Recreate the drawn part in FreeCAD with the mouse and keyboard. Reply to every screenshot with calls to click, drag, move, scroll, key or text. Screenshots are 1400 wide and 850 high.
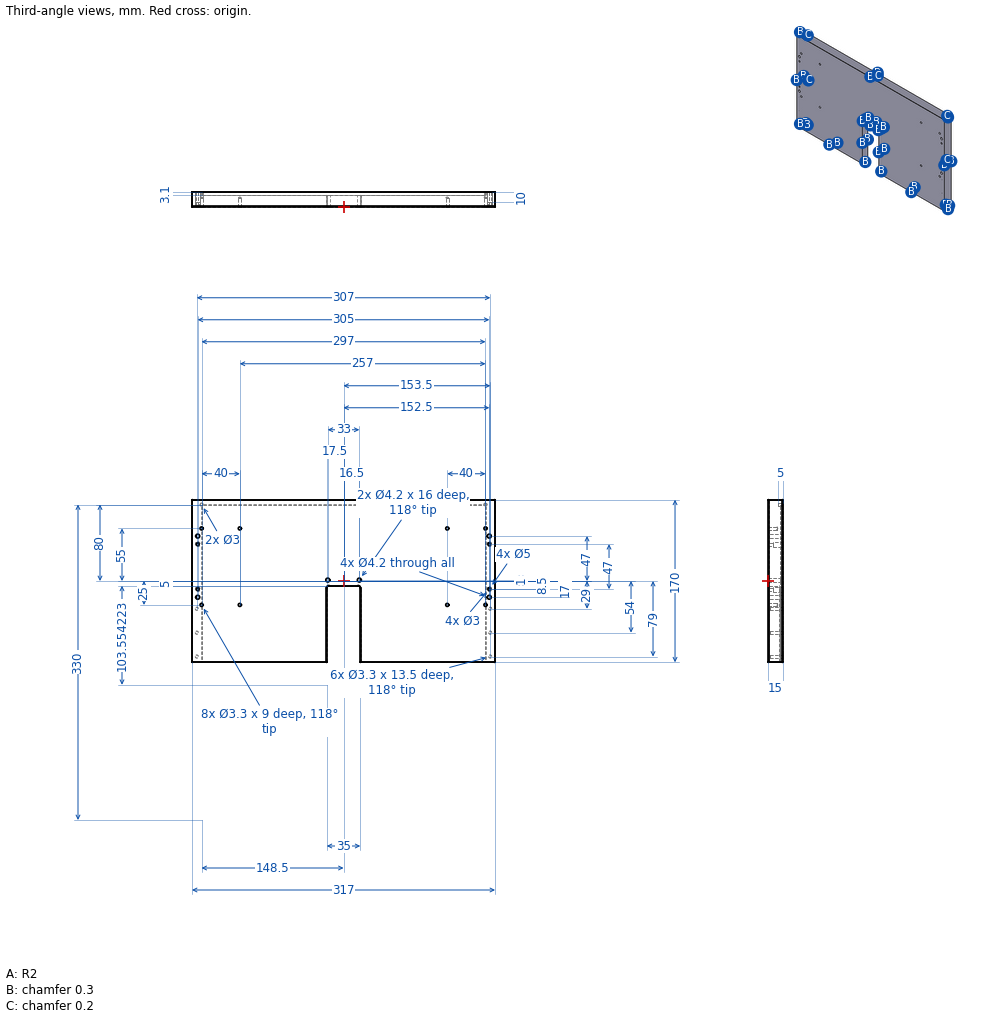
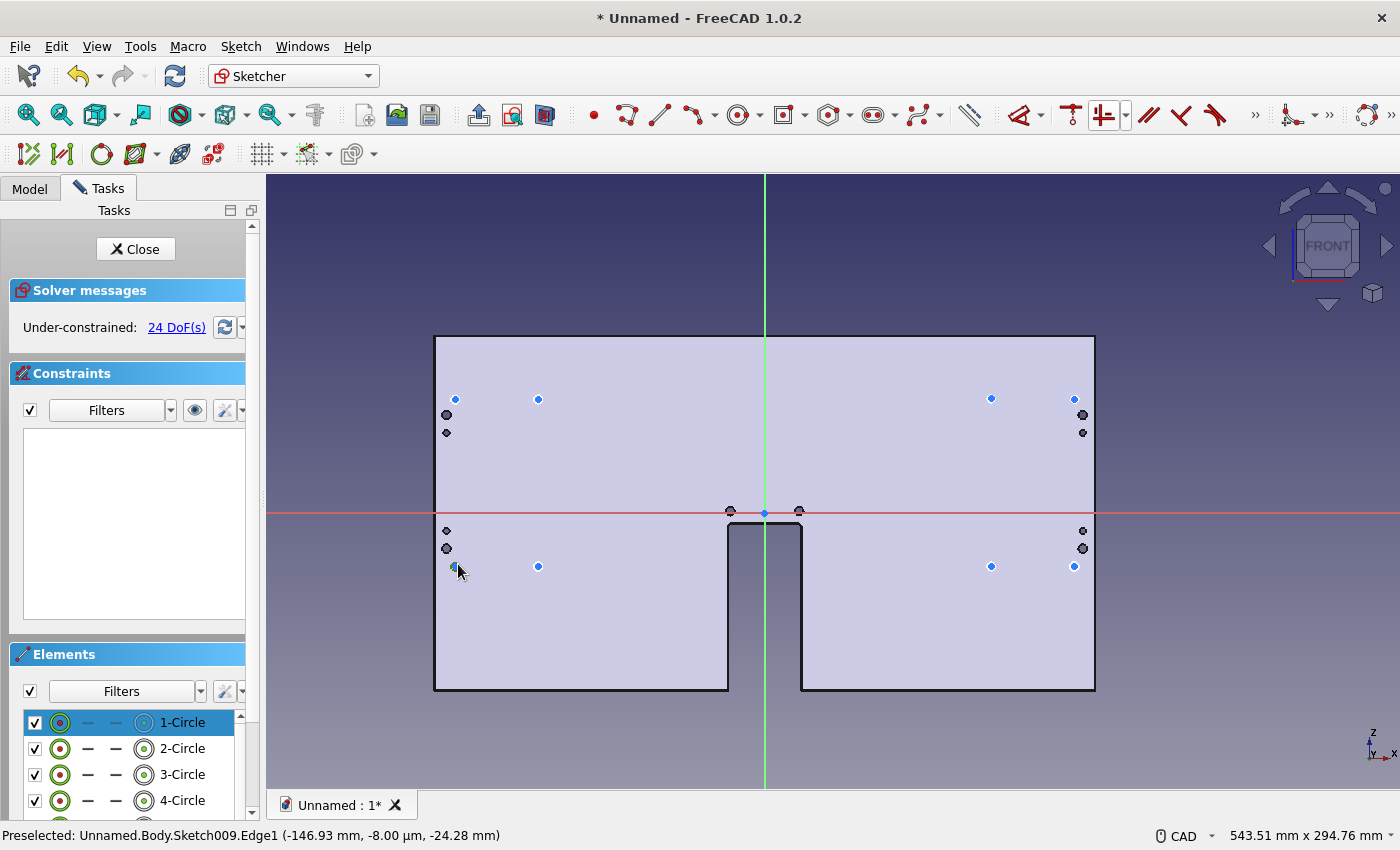
scroll(458, 397, up, 7)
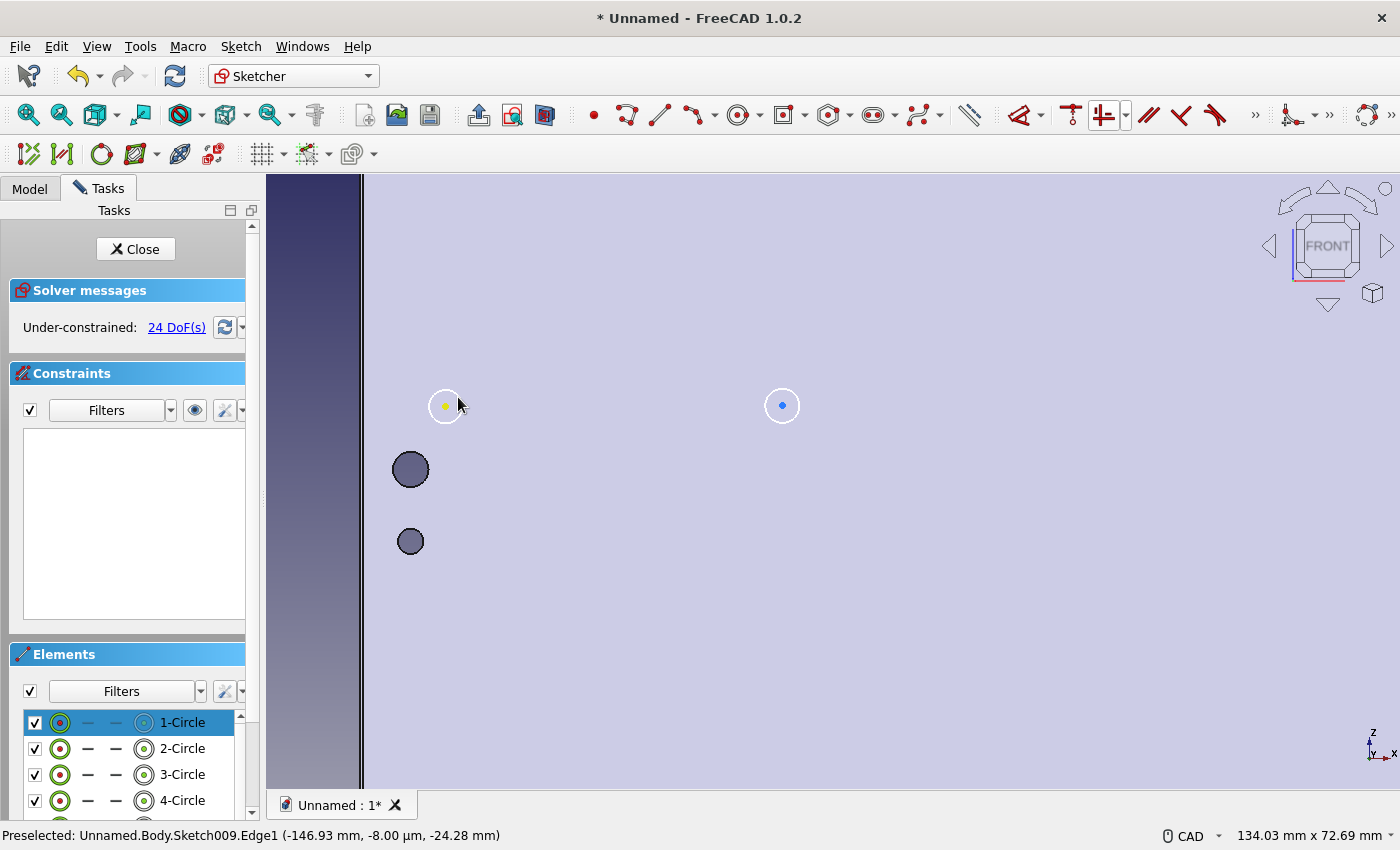
click(458, 395)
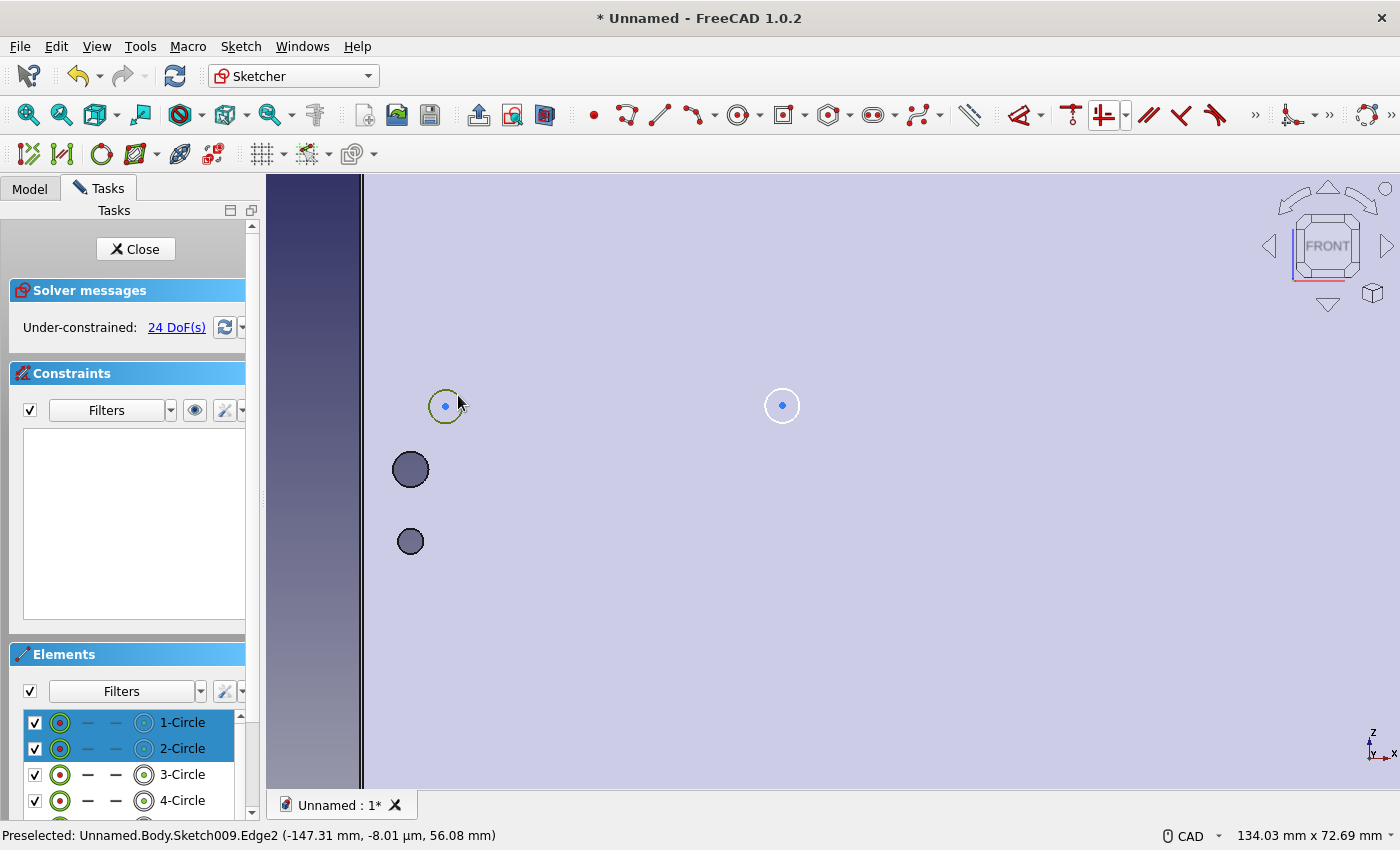
scroll(458, 397, down, 7)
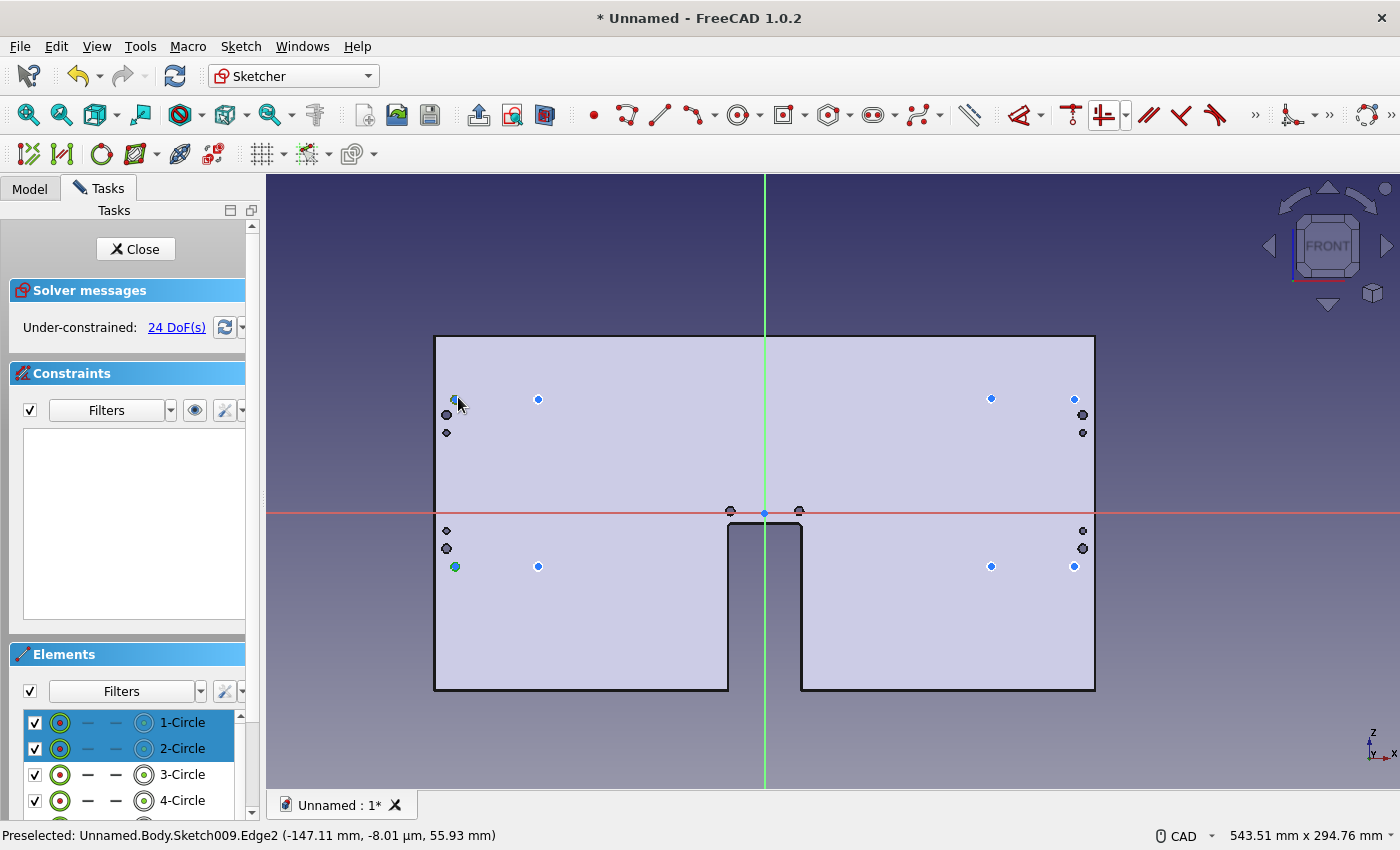
scroll(541, 564, up, 6)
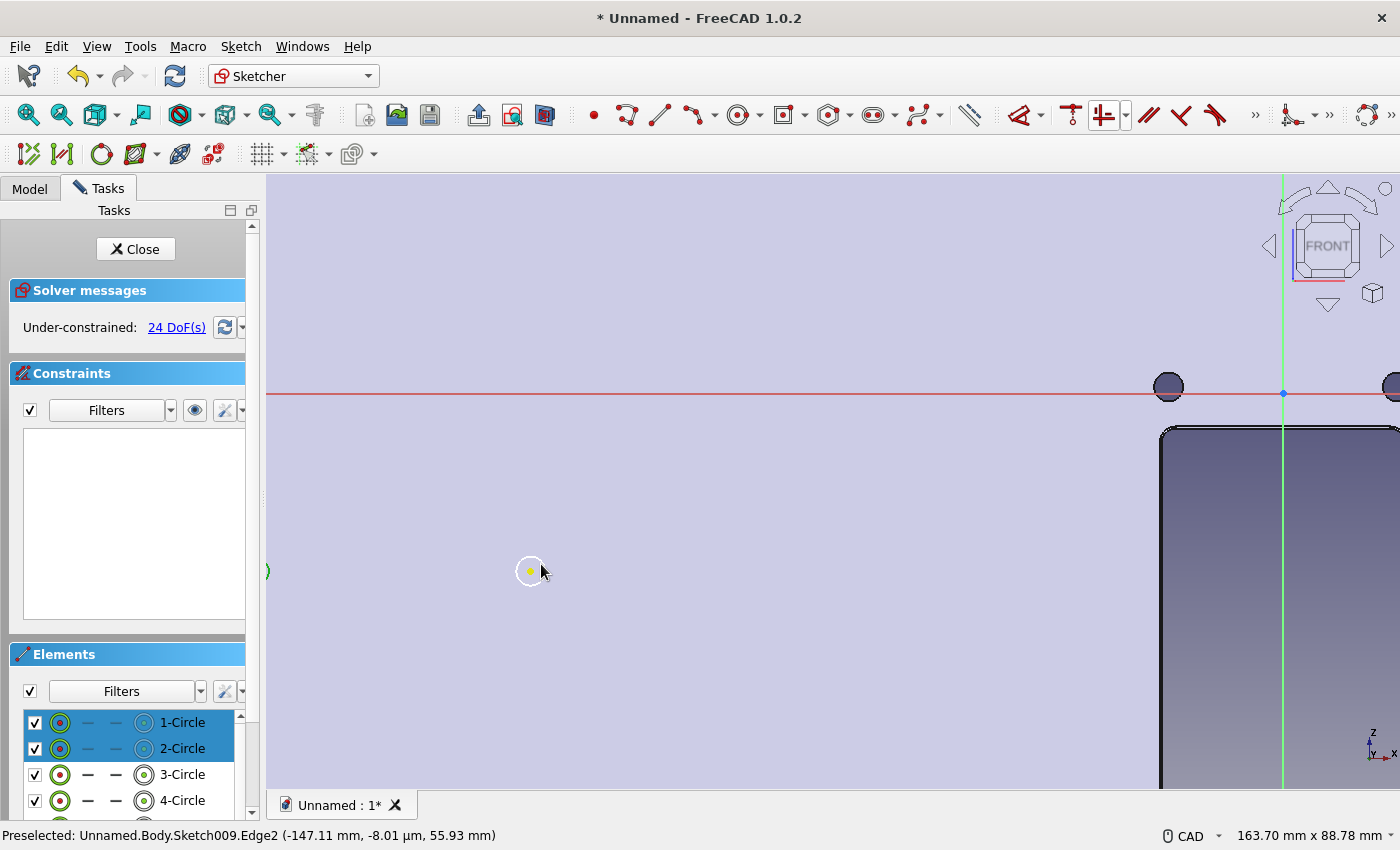
click(541, 561)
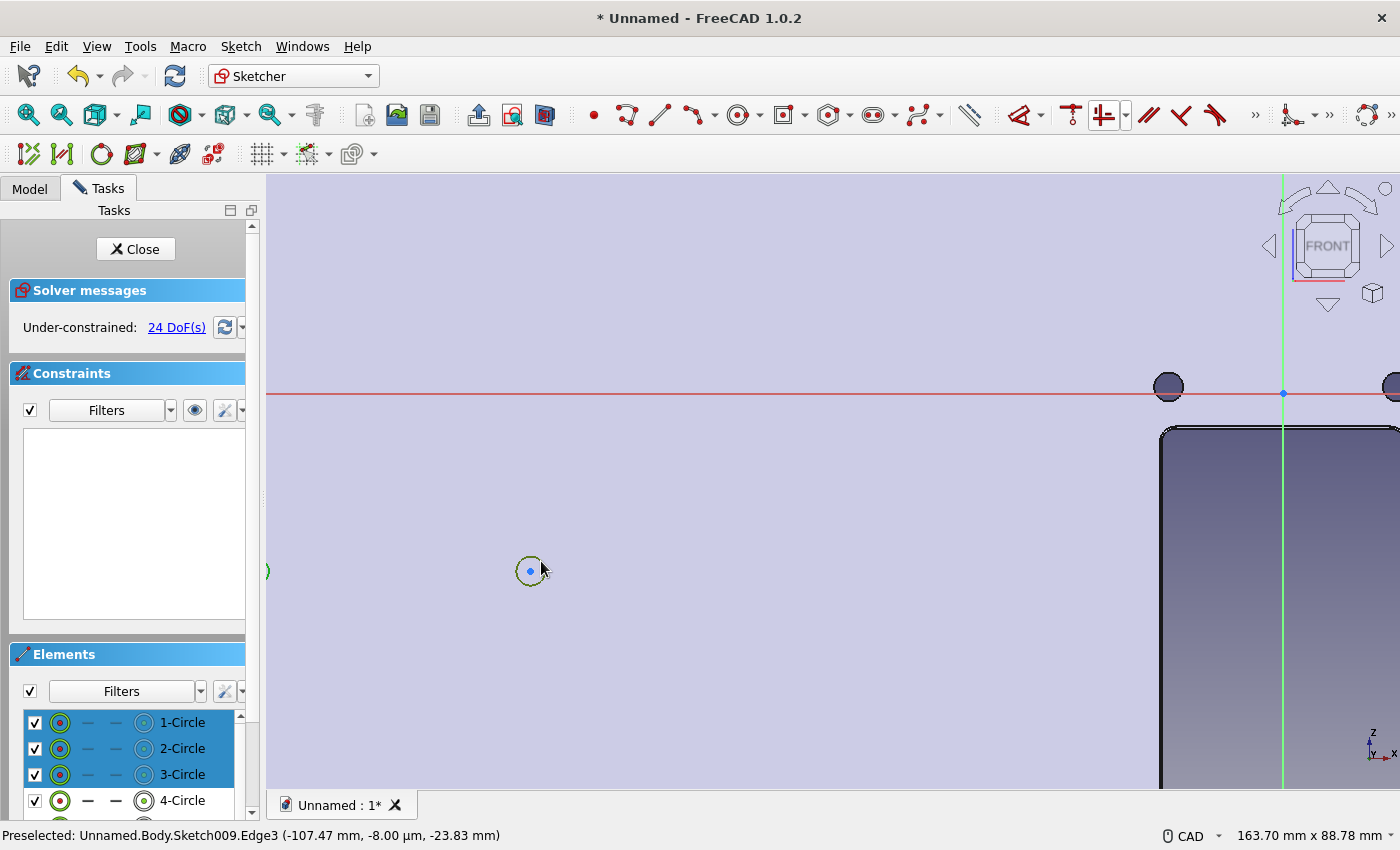
scroll(541, 564, down, 6)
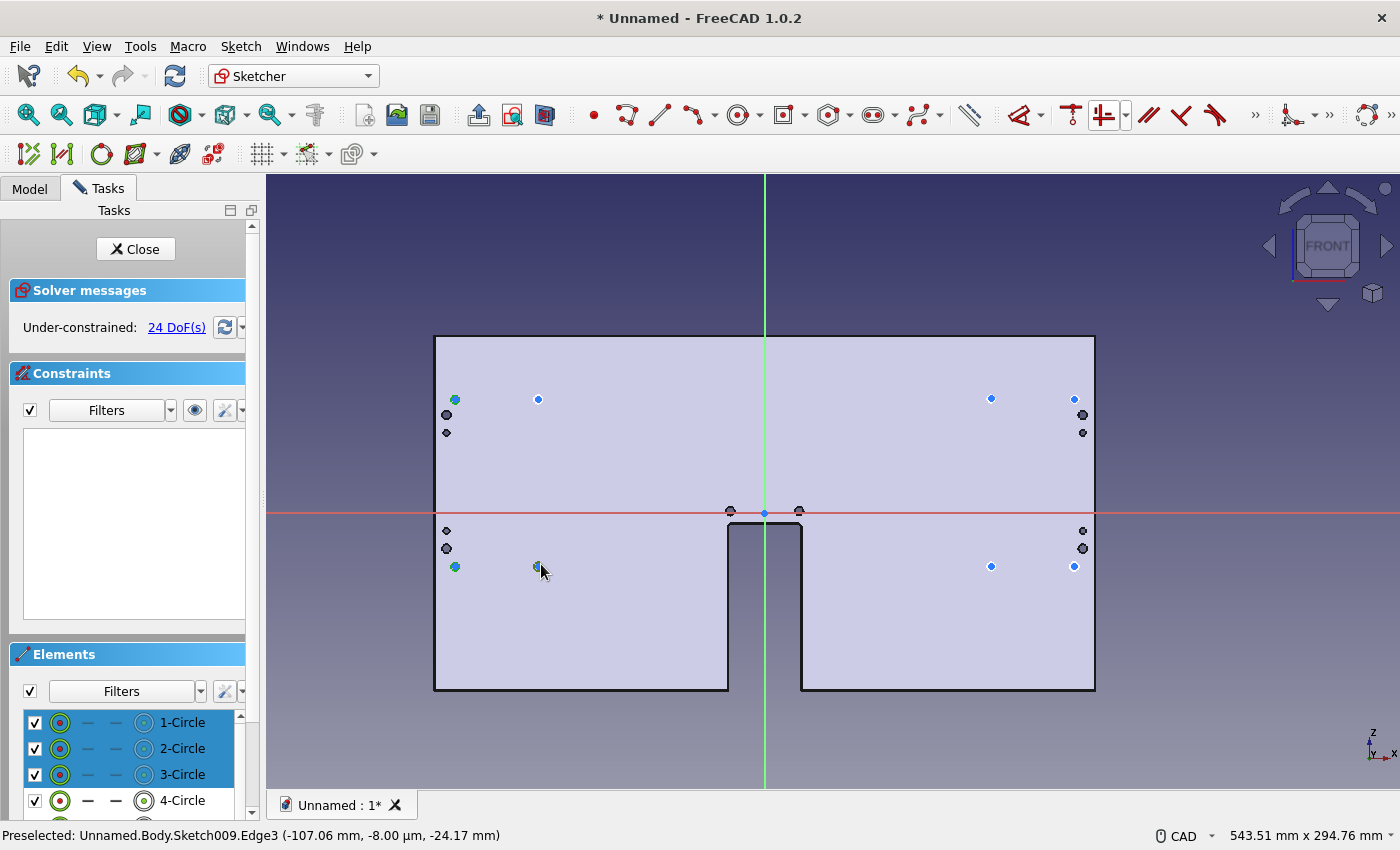
scroll(541, 396, up, 6)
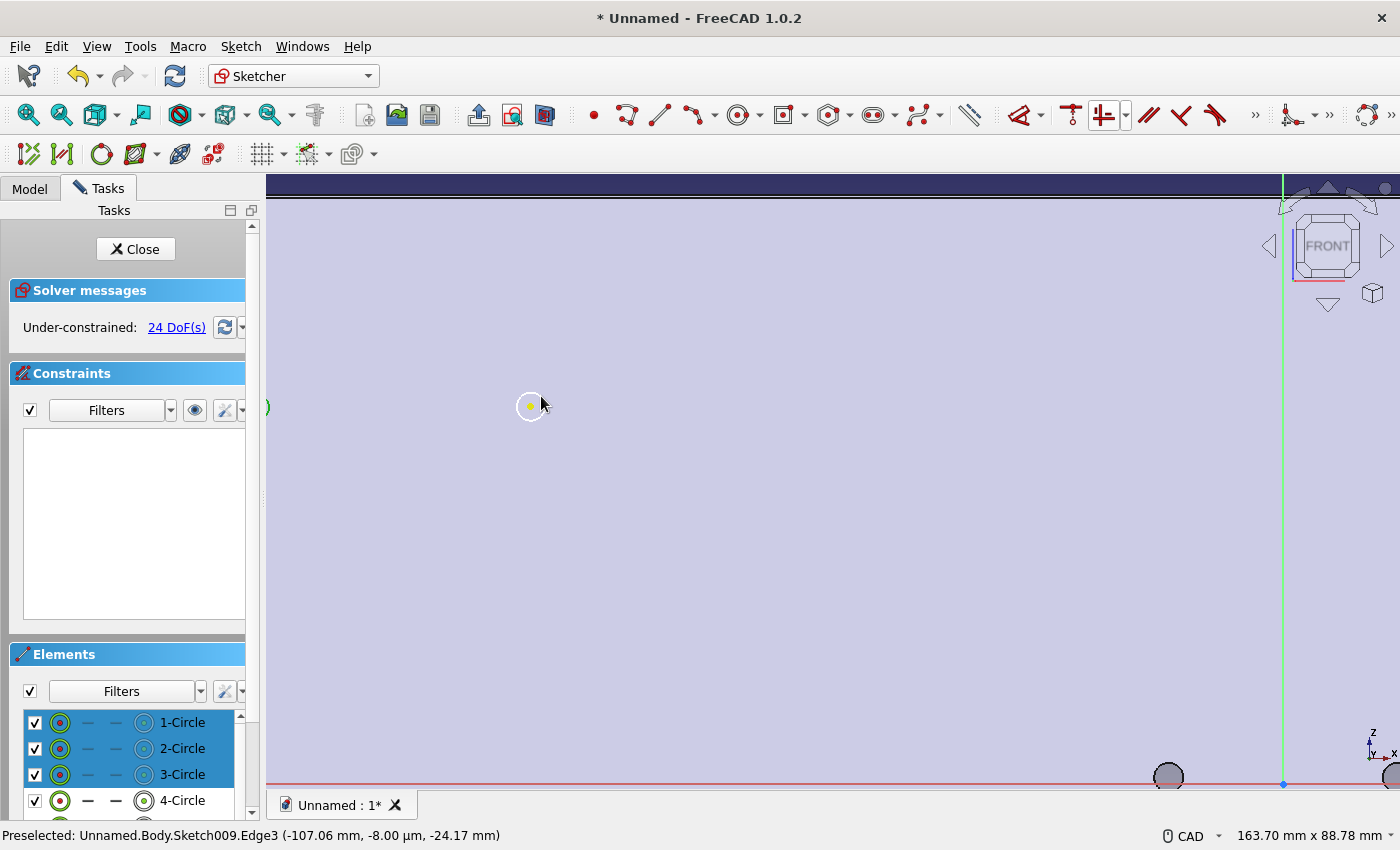
click(541, 397)